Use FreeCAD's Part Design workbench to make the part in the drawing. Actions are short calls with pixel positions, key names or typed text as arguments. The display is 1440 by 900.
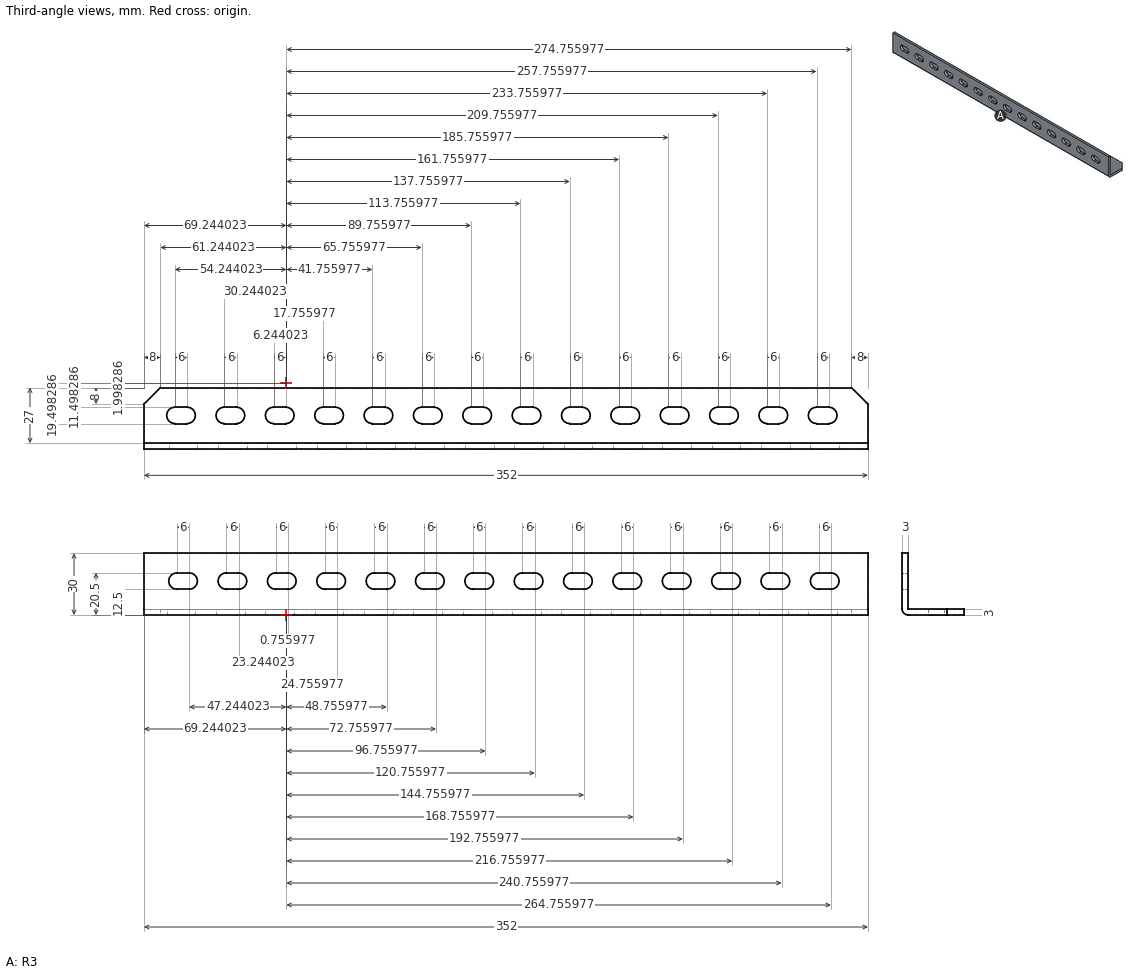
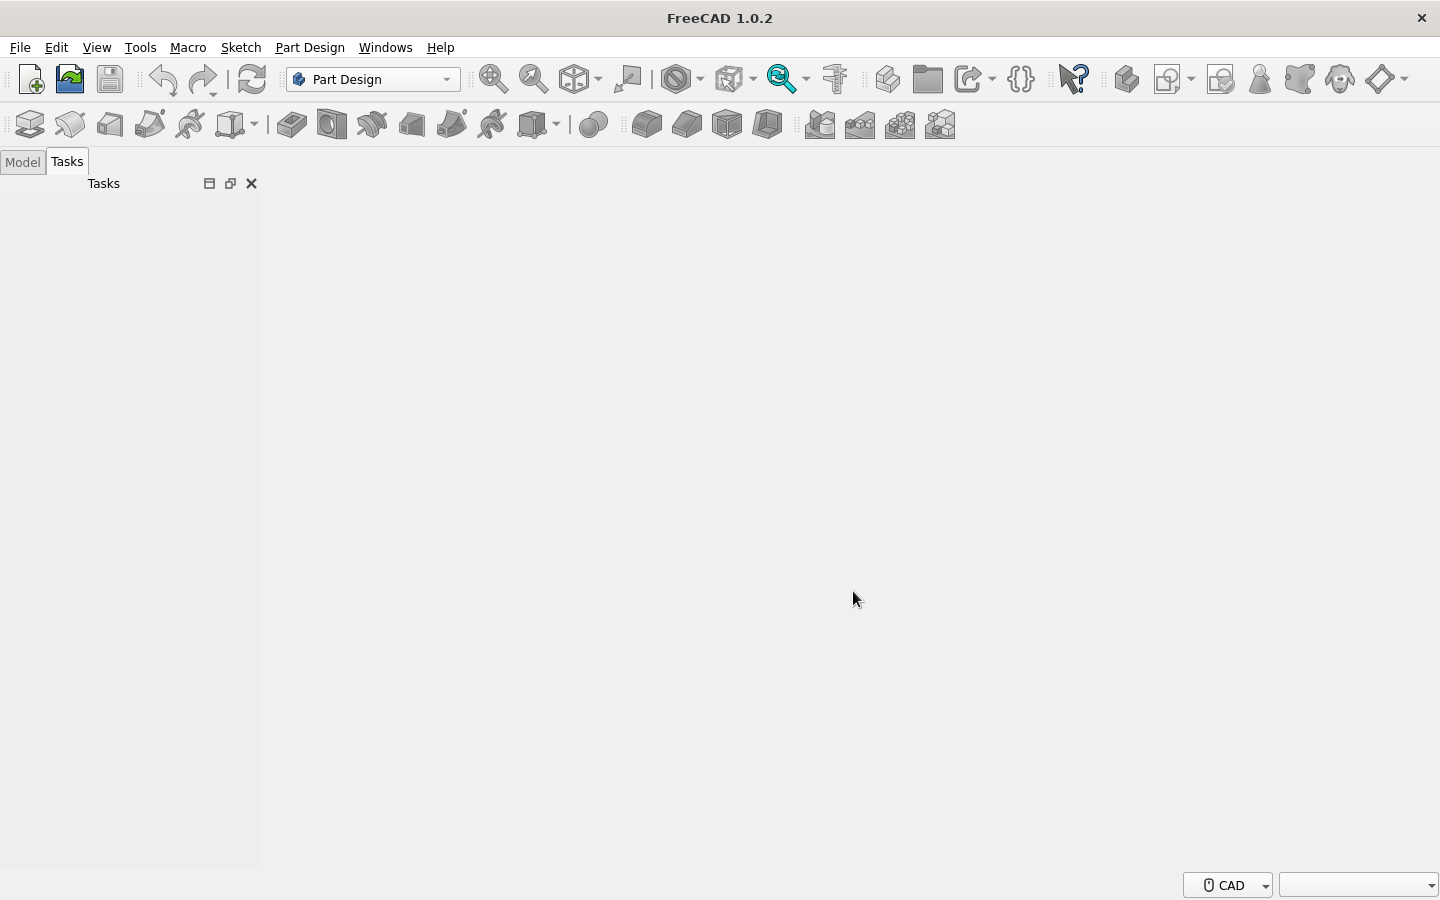
click(30, 80)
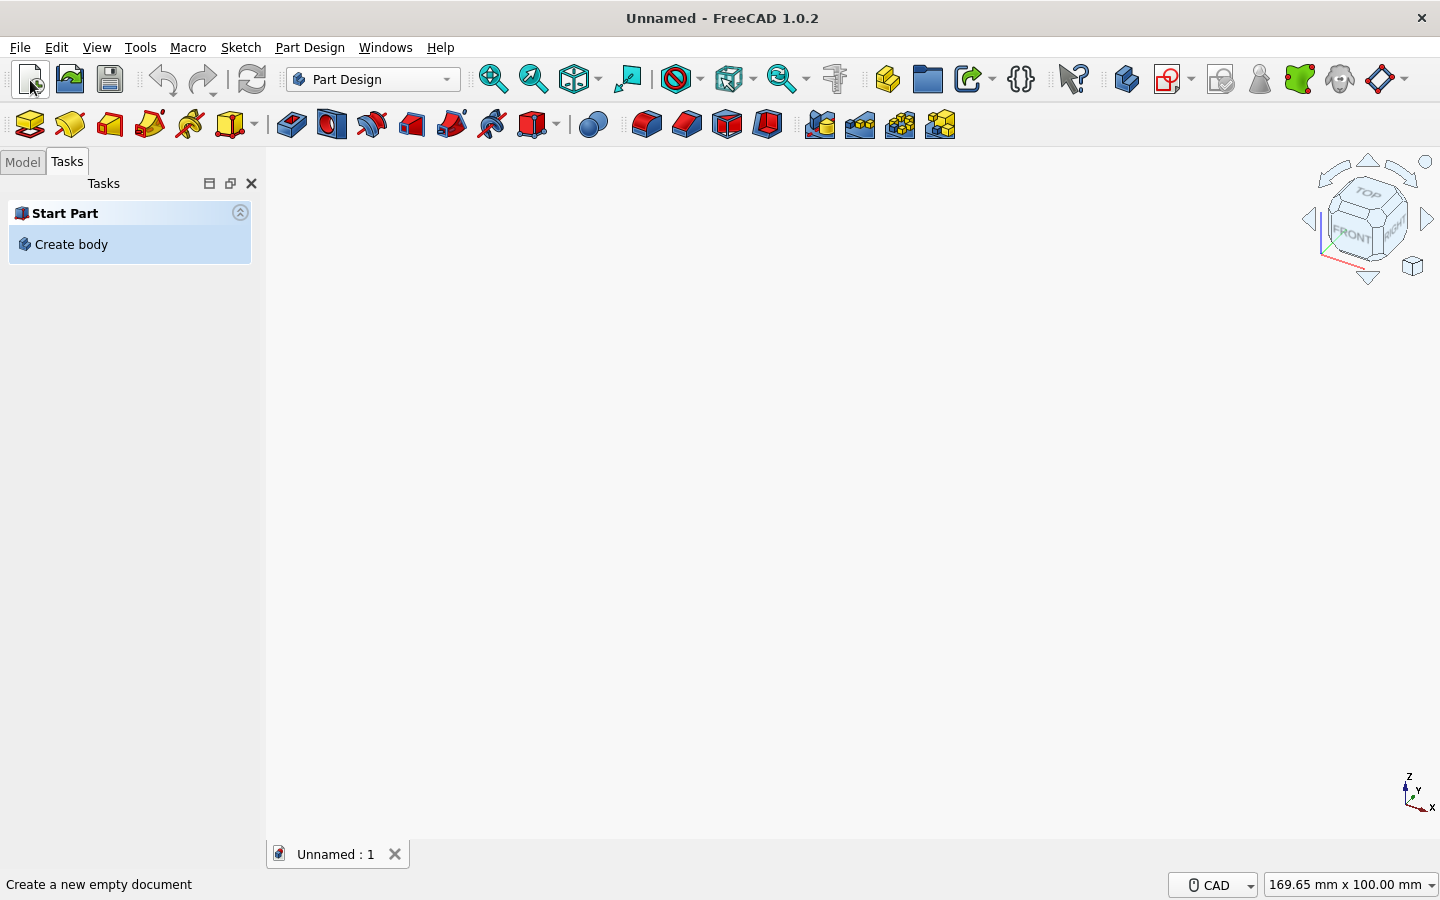
click(1168, 80)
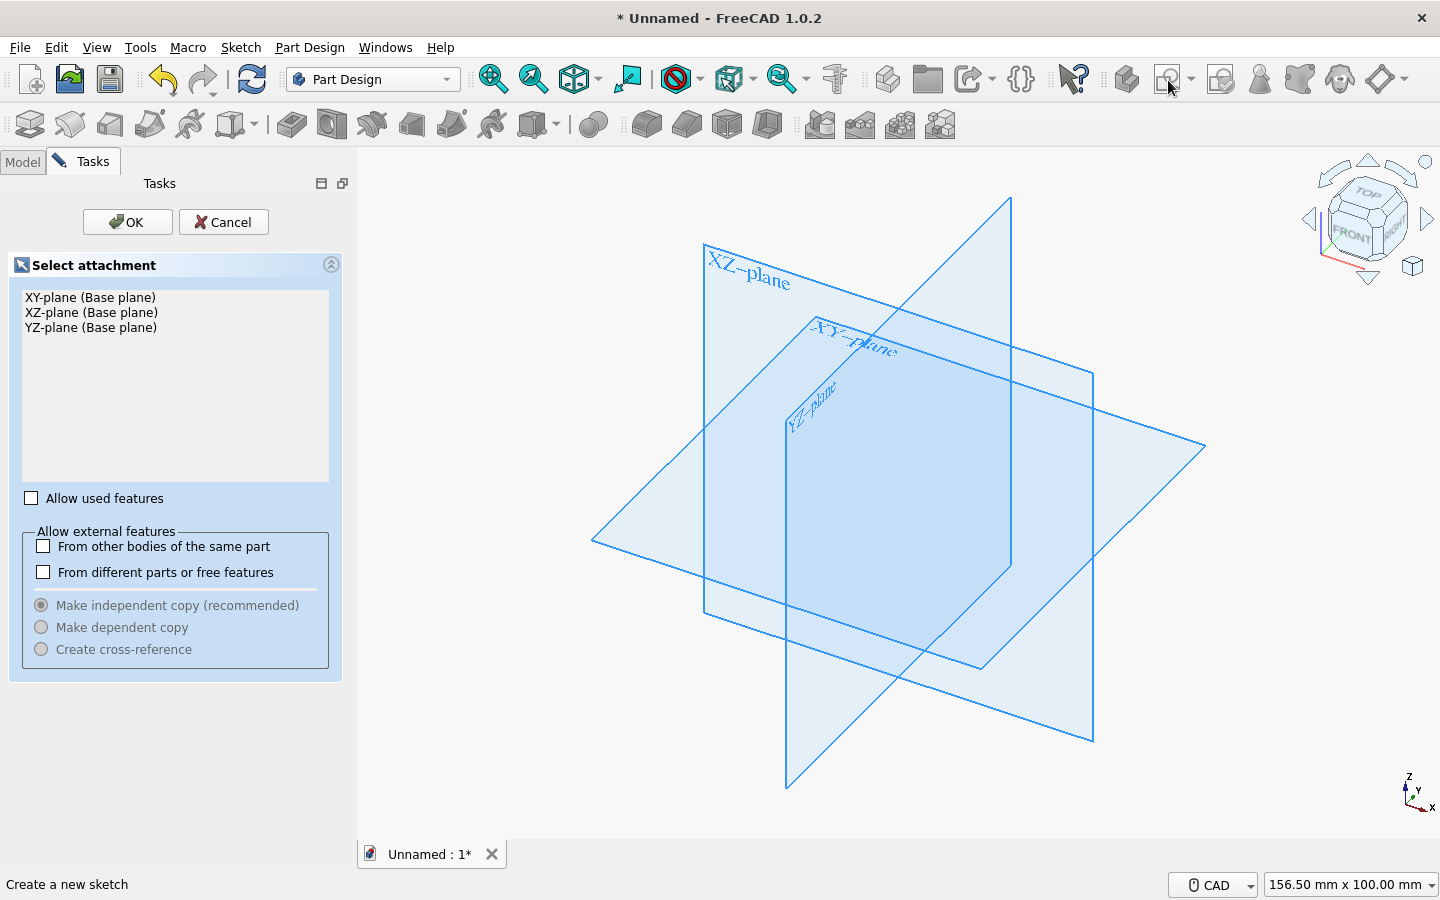
click(82, 298)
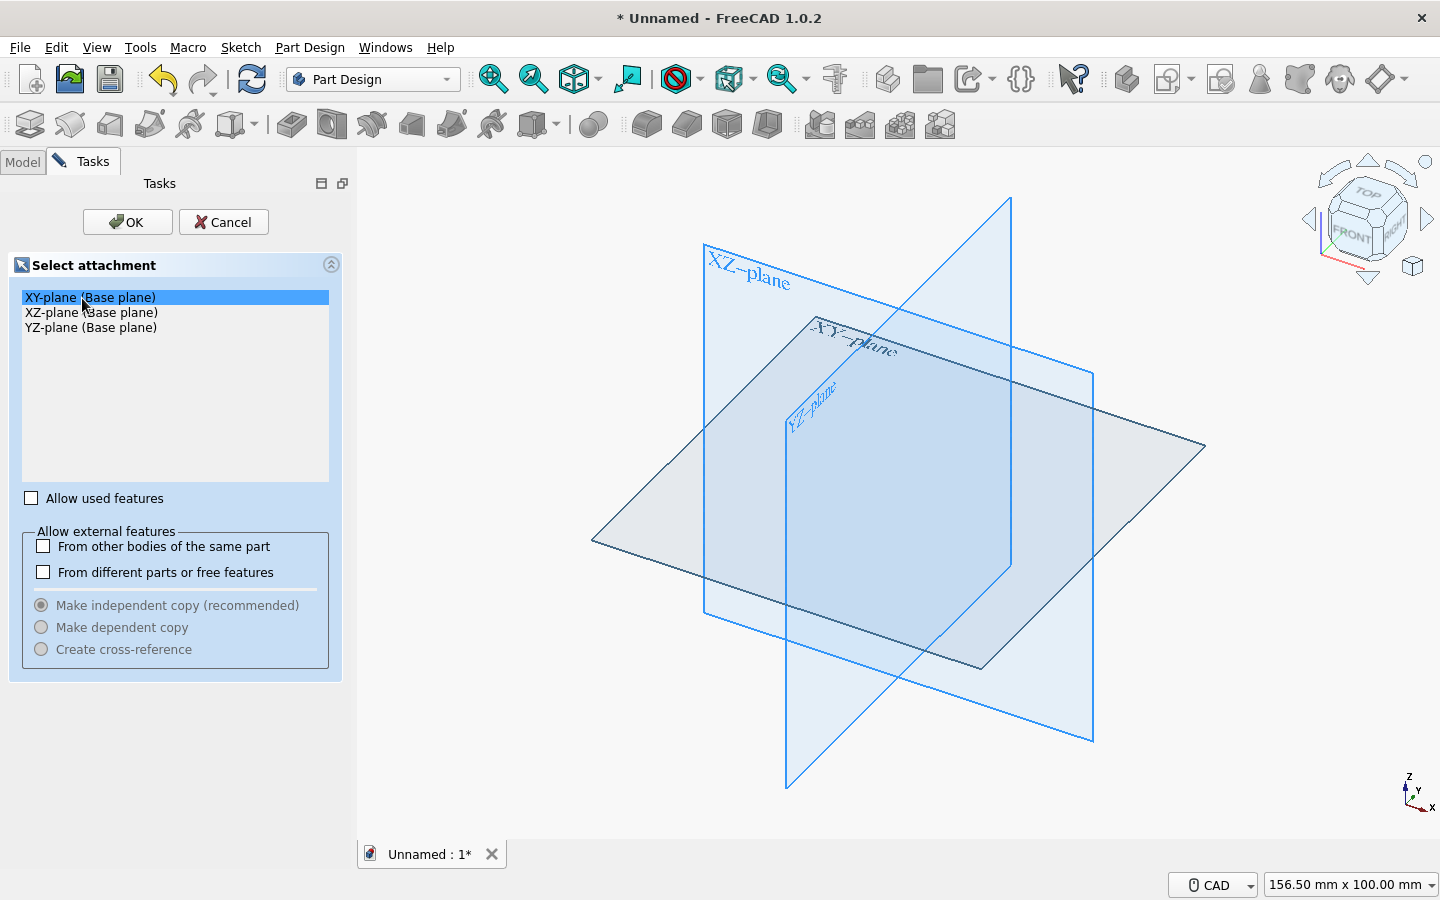
click(128, 222)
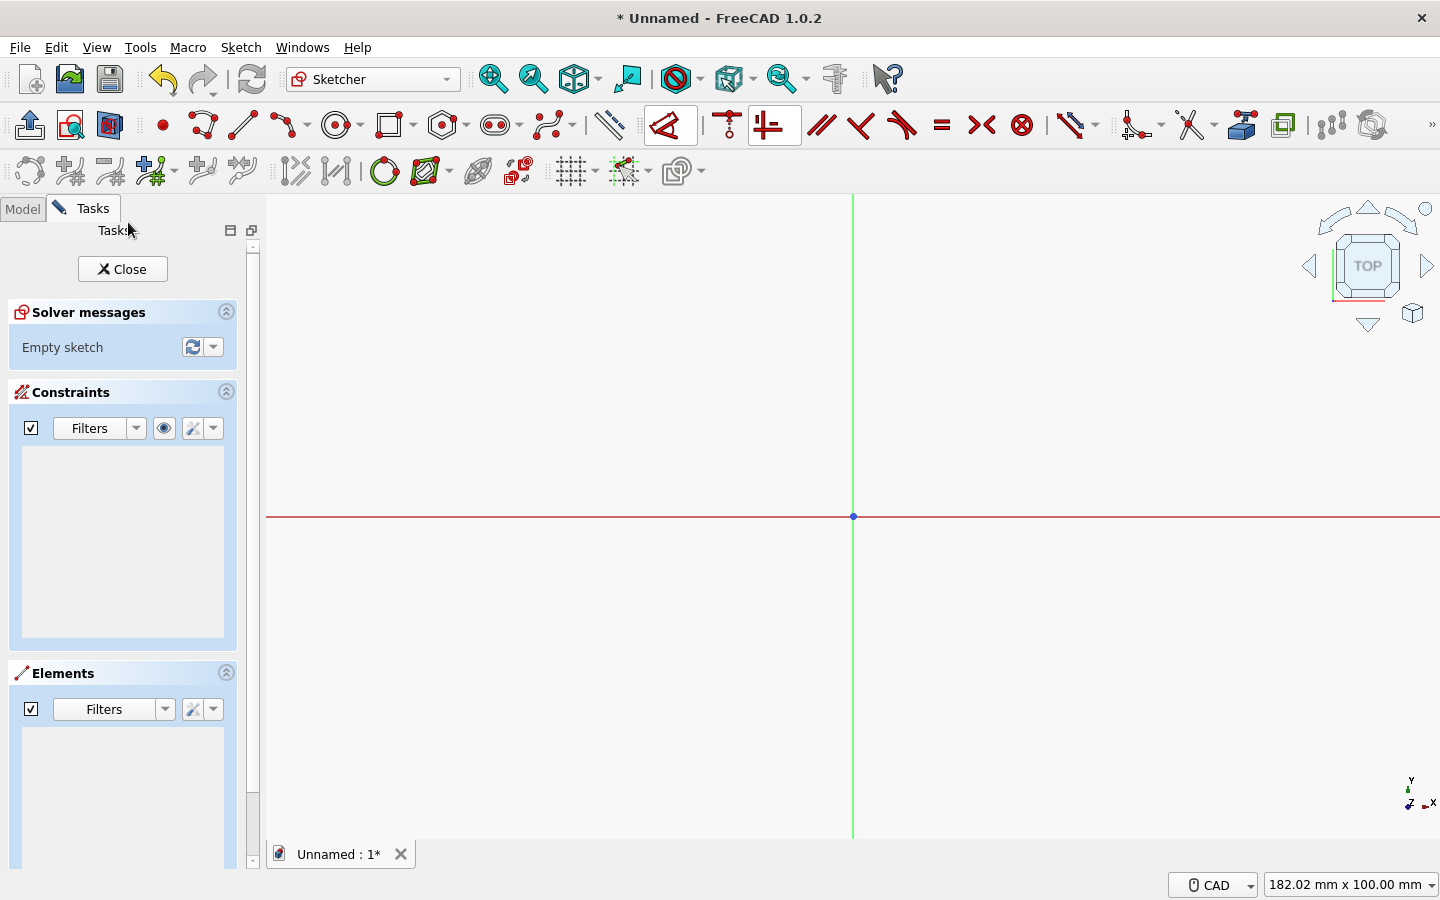
scroll(458, 476, down, 6)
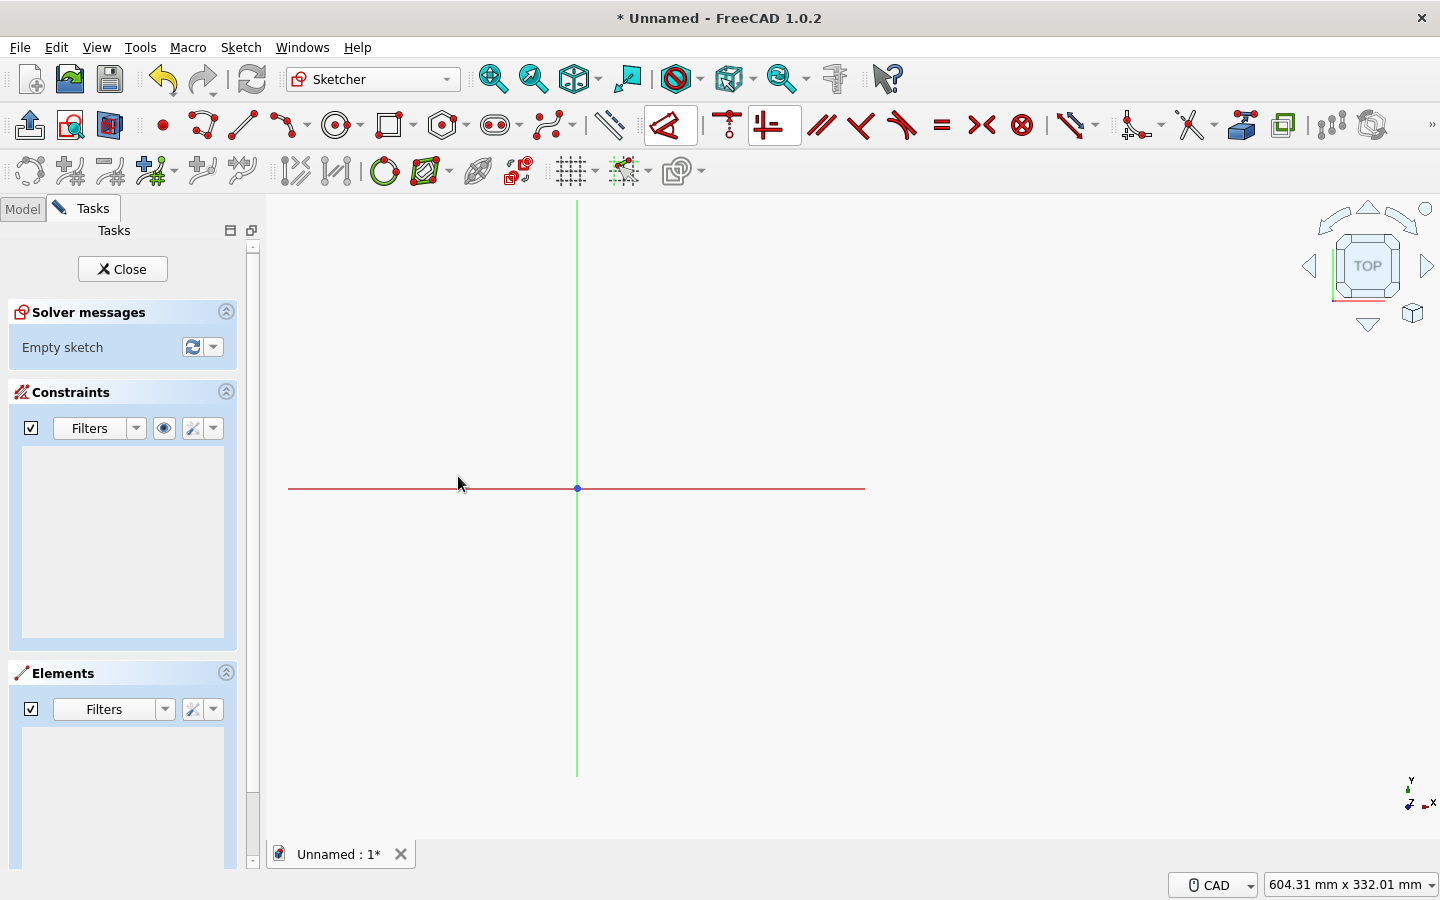
click(390, 126)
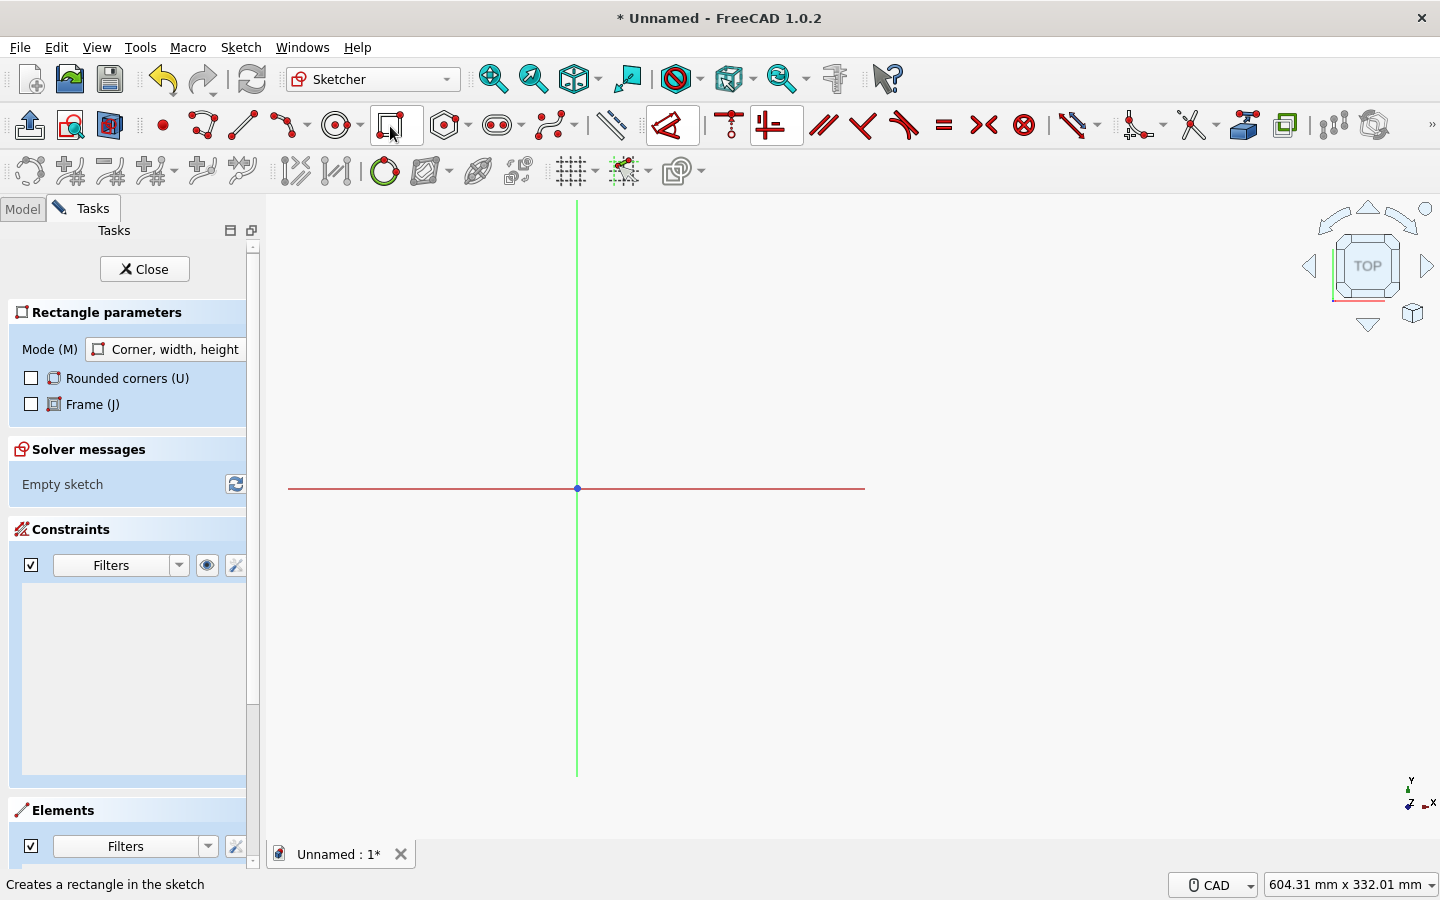
scroll(443, 492, up, 8)